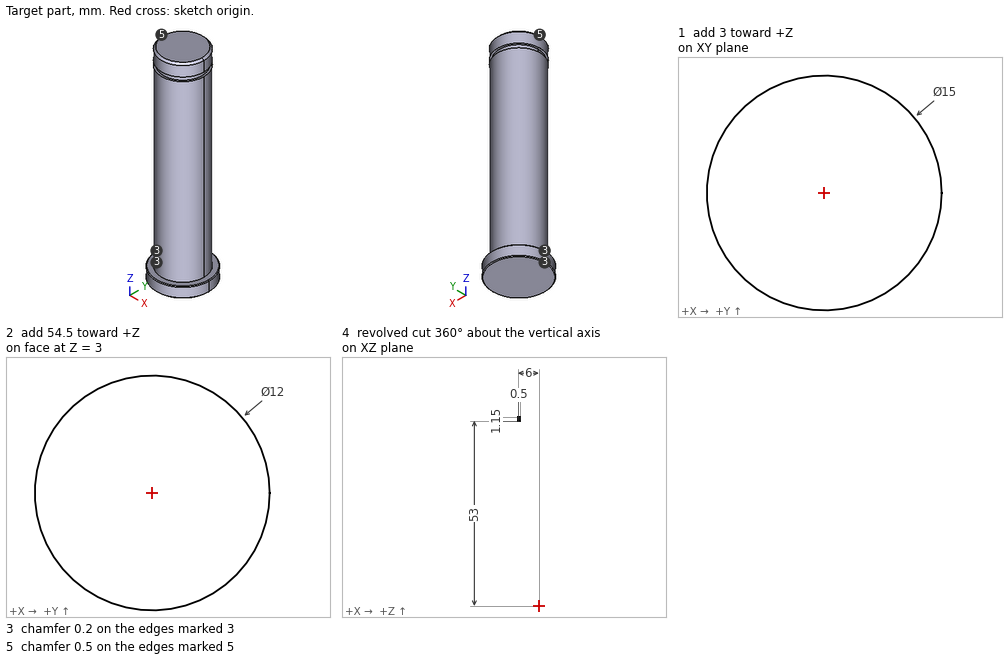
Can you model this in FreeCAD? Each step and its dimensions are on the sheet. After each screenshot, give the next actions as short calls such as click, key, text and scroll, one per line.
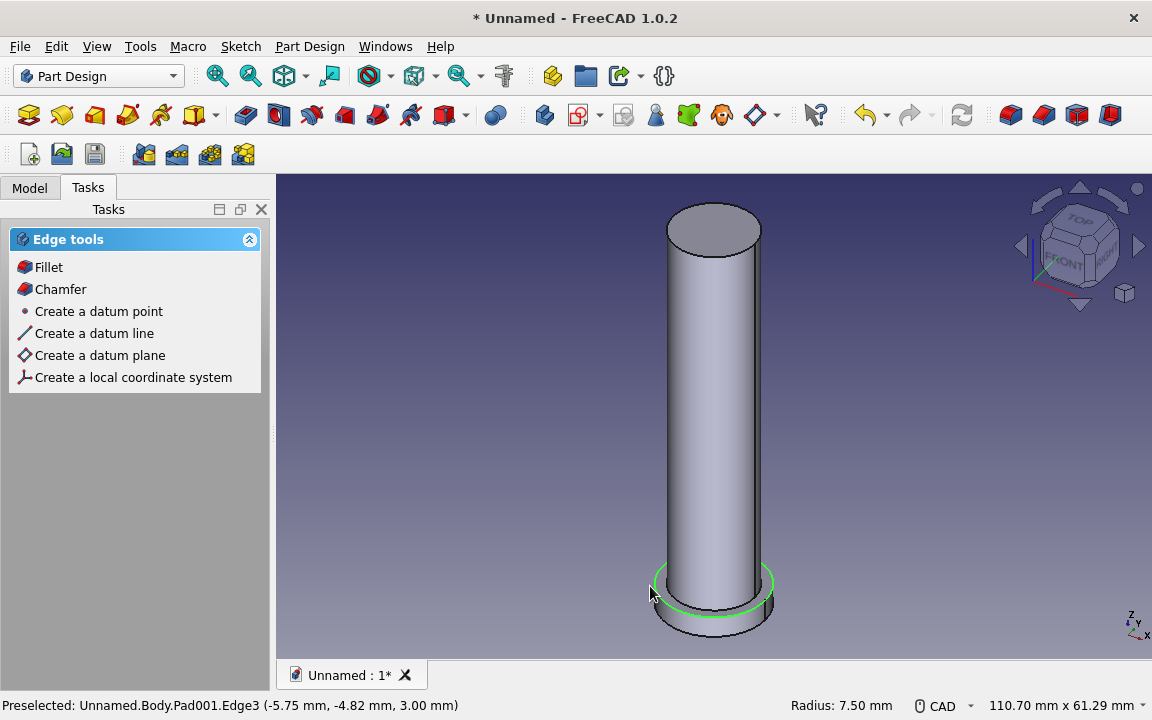
key(0)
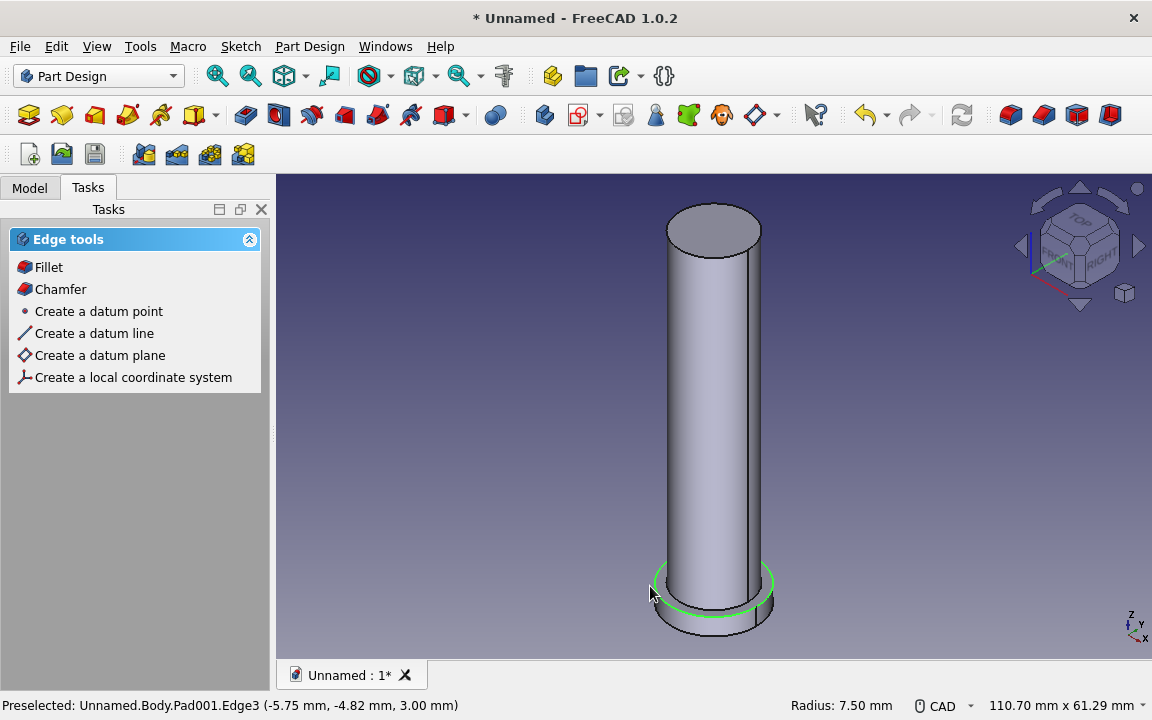
key(2)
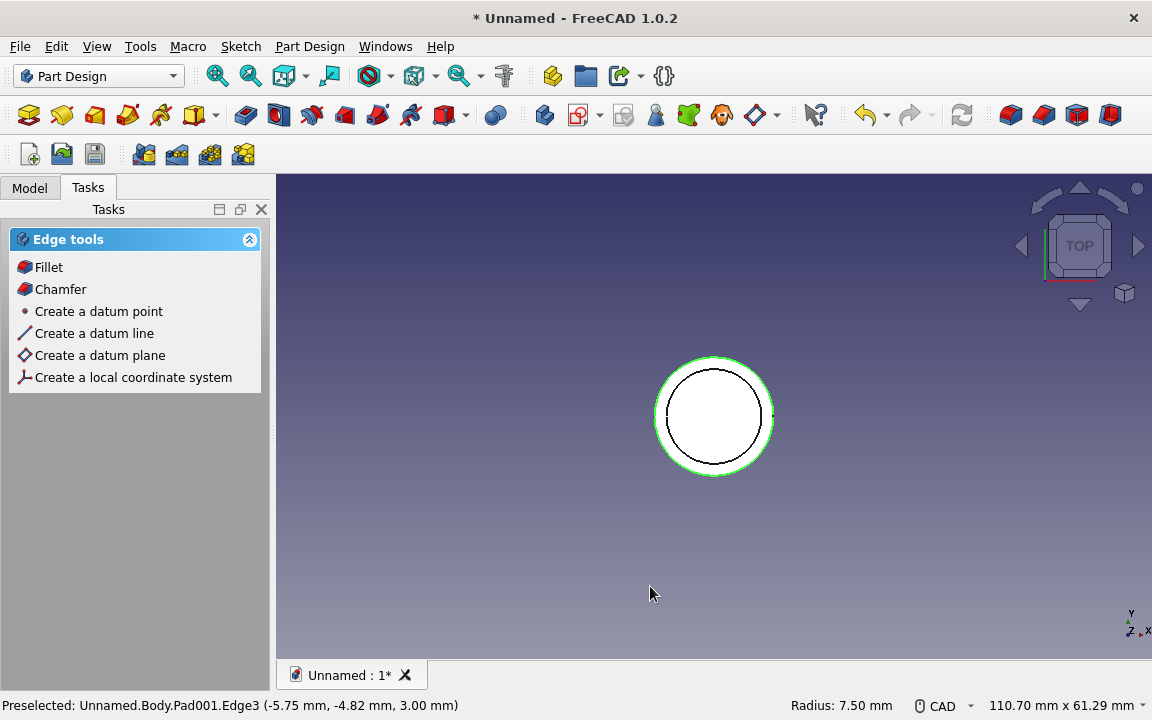
click(218, 76)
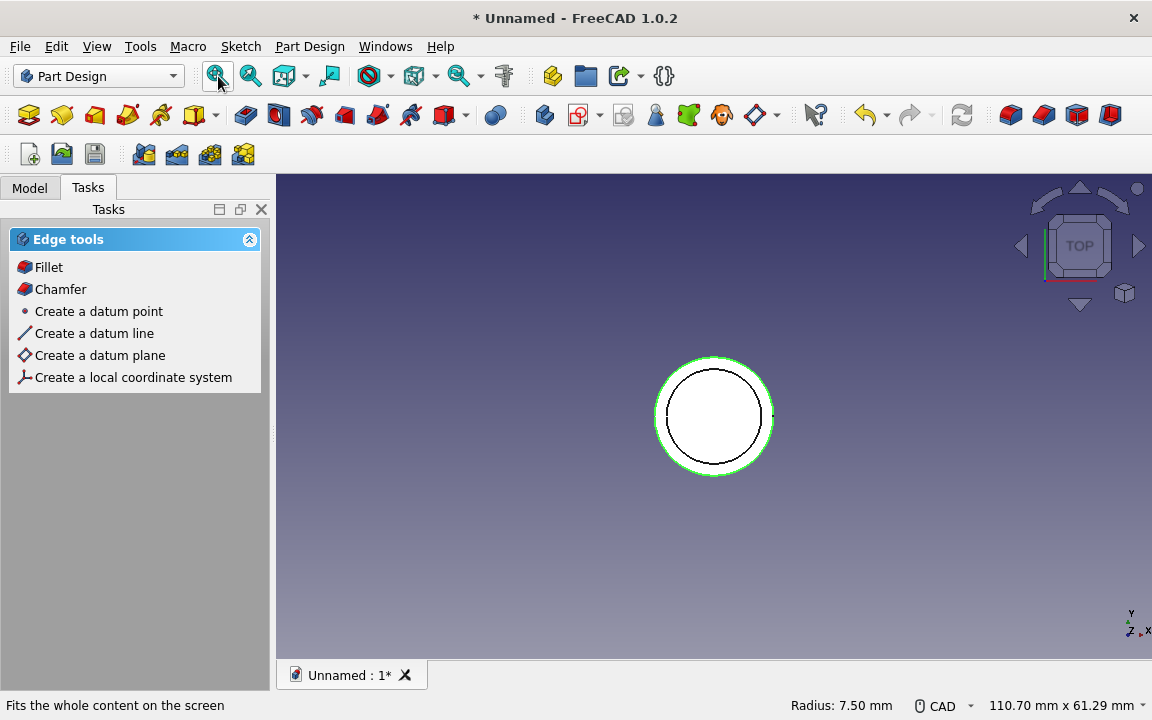
key(1)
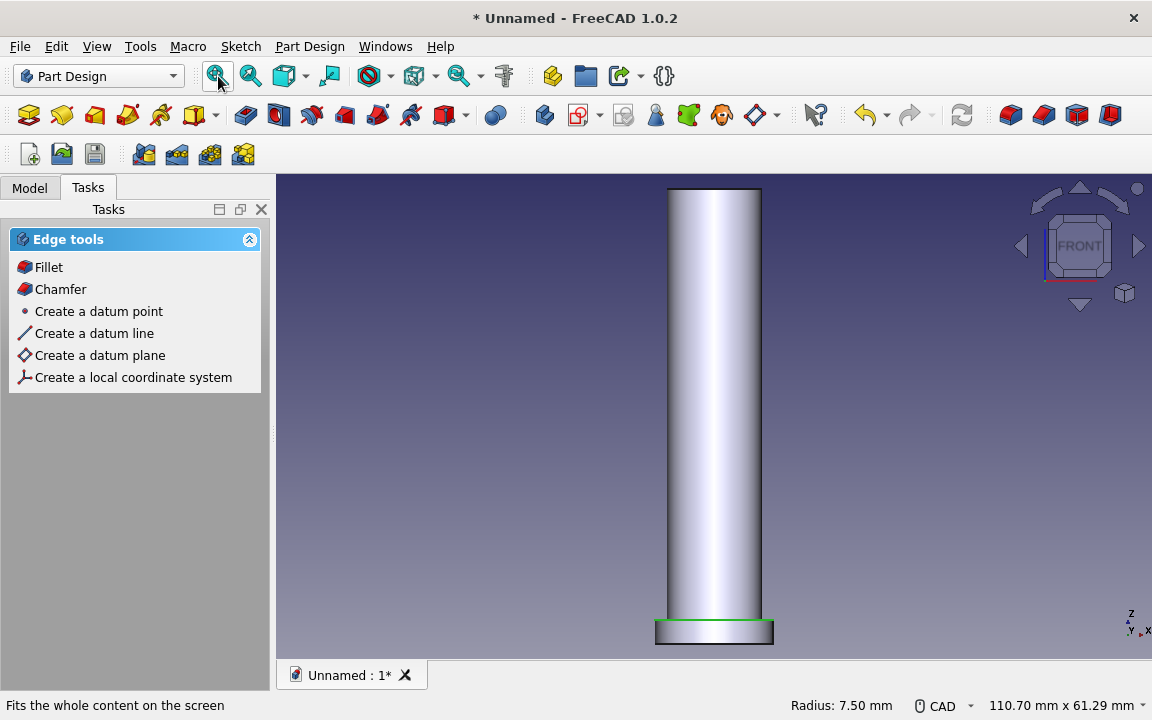
key(3)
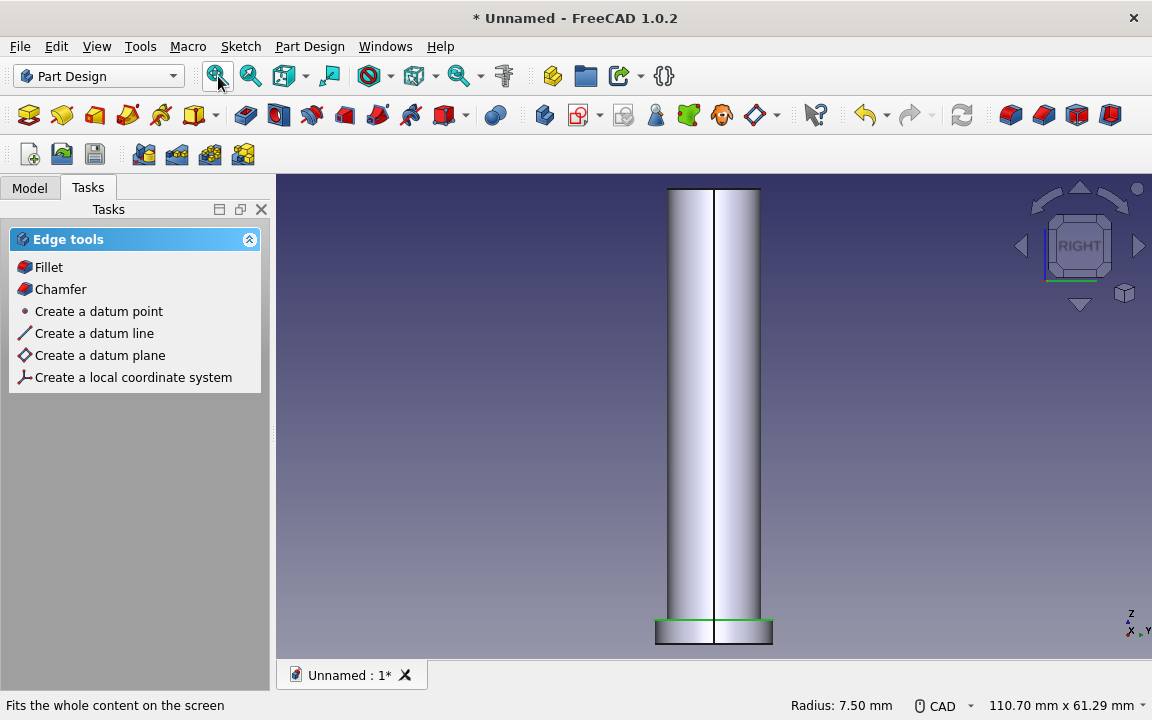
key(5)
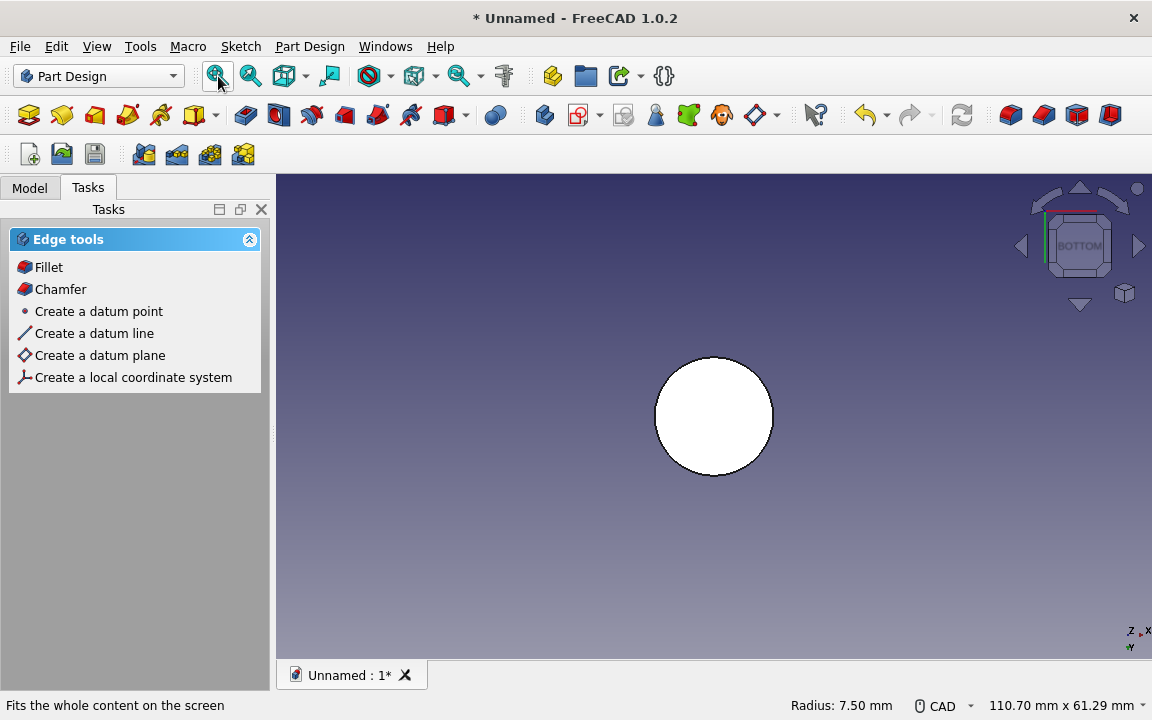
click(218, 76)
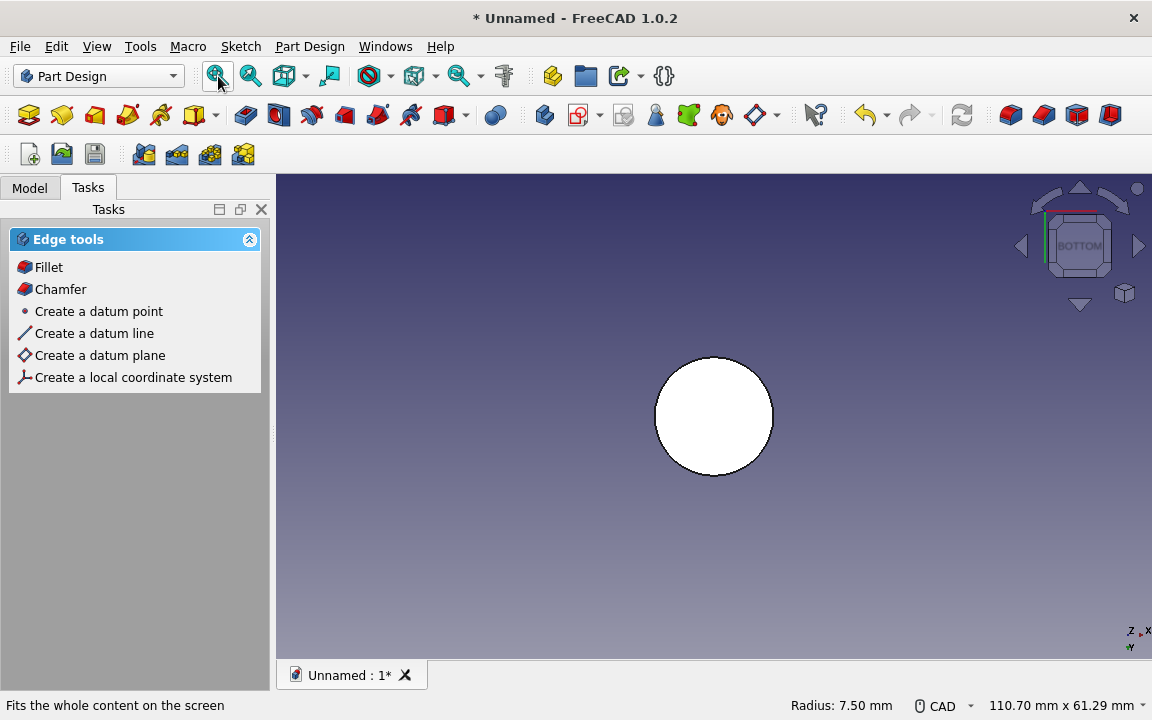
click(696, 472, ctrl)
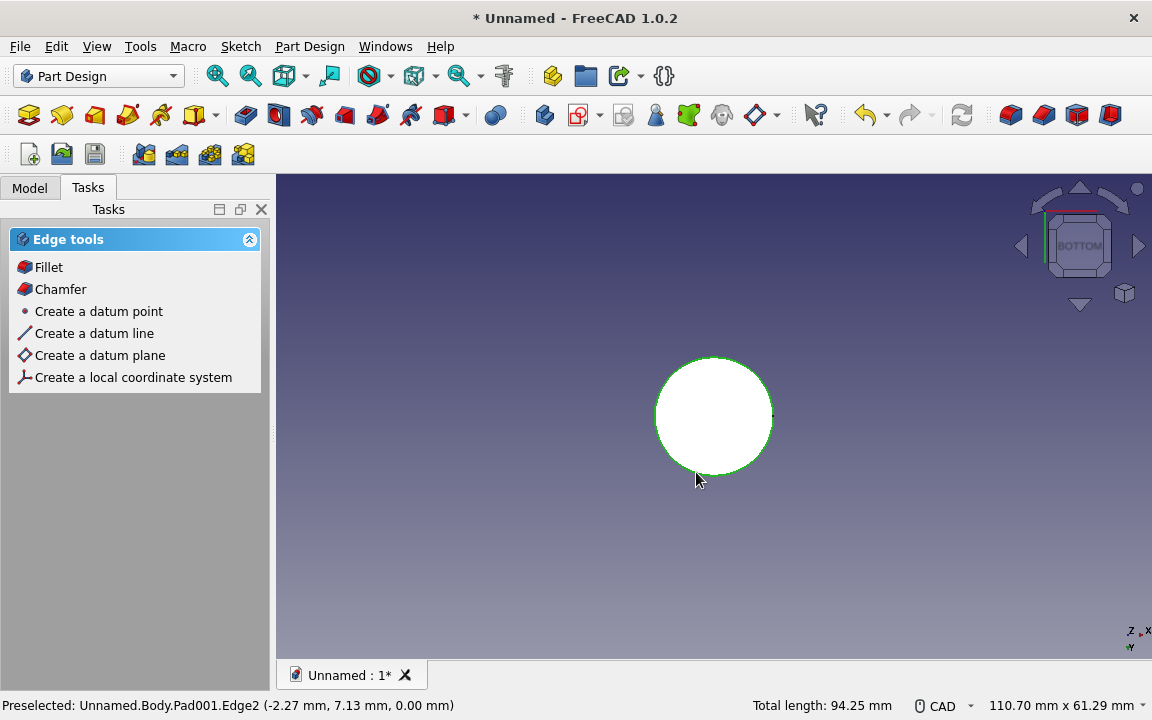
click(1044, 116)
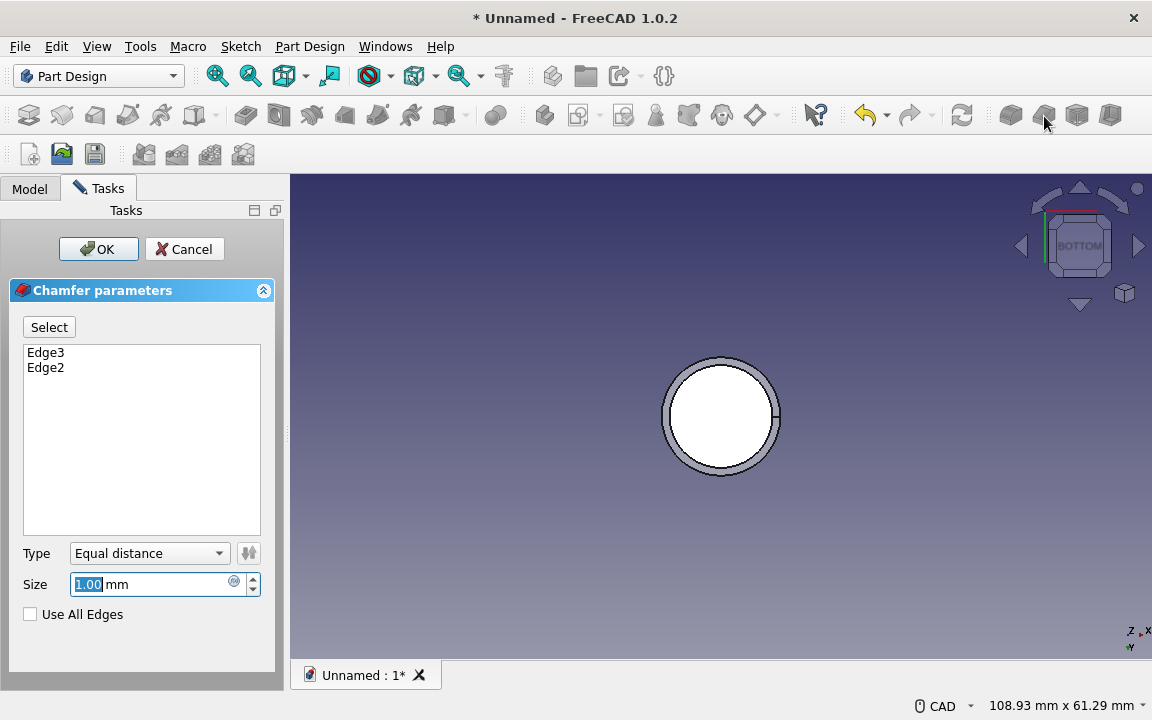
text(0.2)
key(Tab)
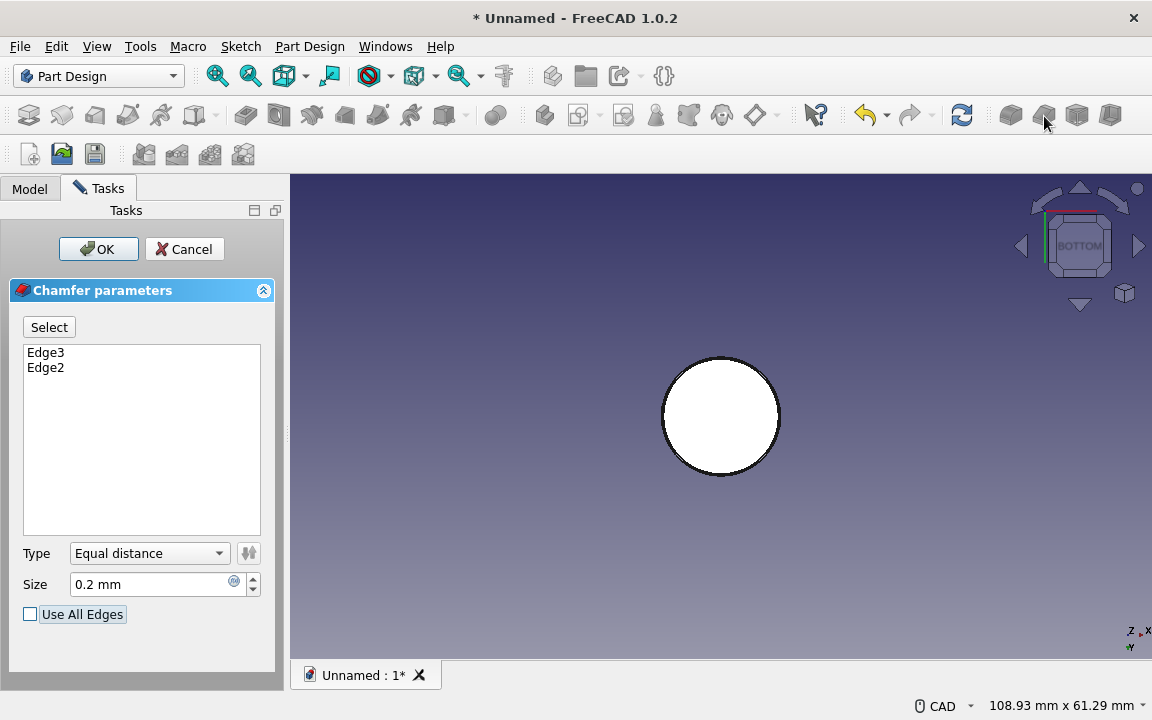
click(99, 249)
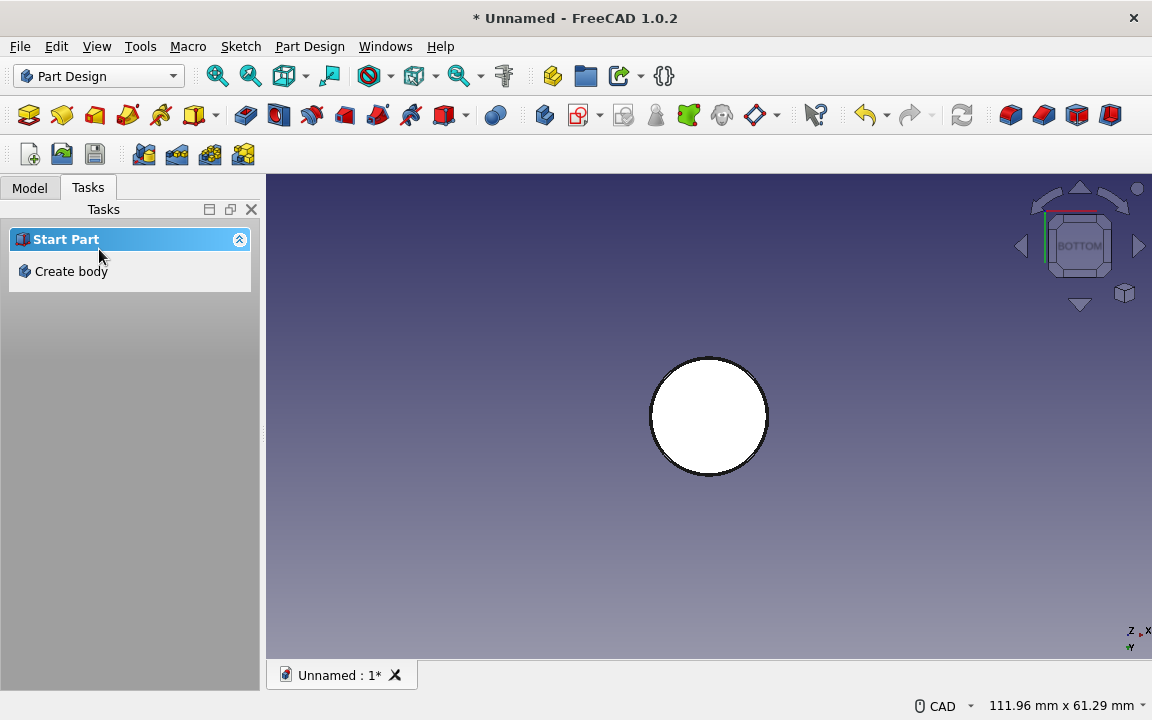
key(v)
key(f)